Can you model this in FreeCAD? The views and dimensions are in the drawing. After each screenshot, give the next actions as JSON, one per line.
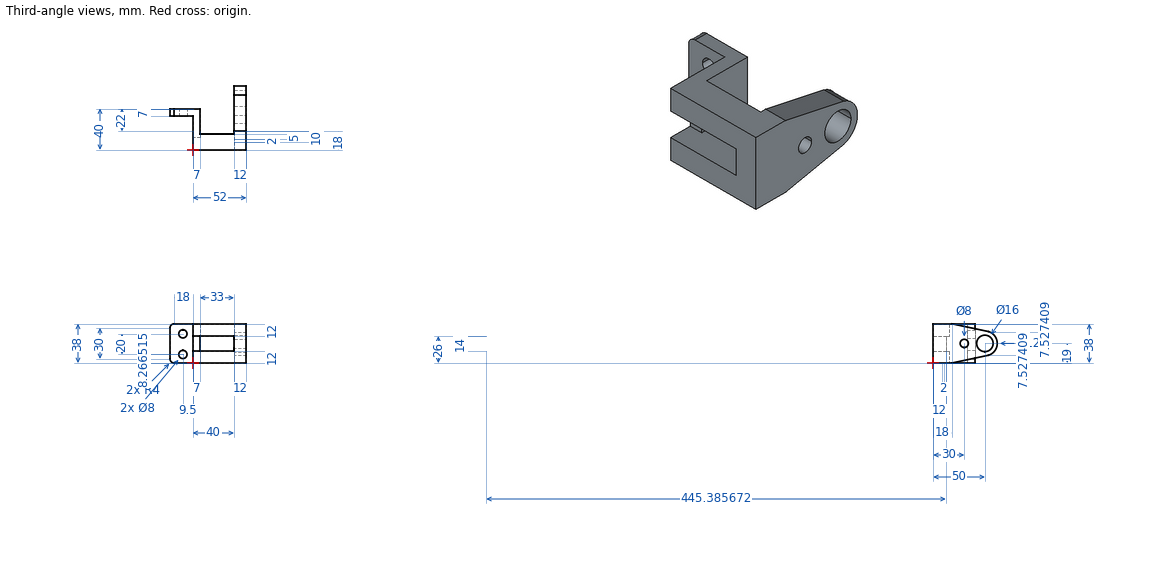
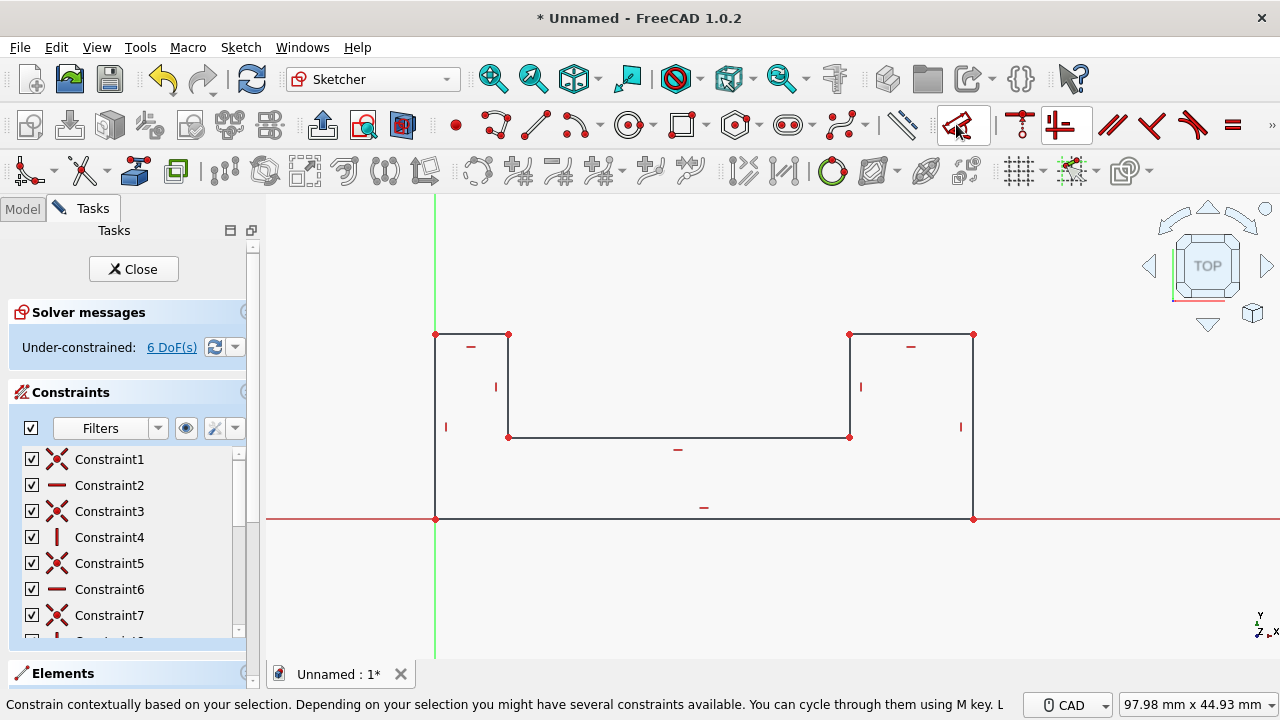
{"action": "left_click", "coordinate": [486, 334]}
{"action": "left_click", "coordinate": [472, 300]}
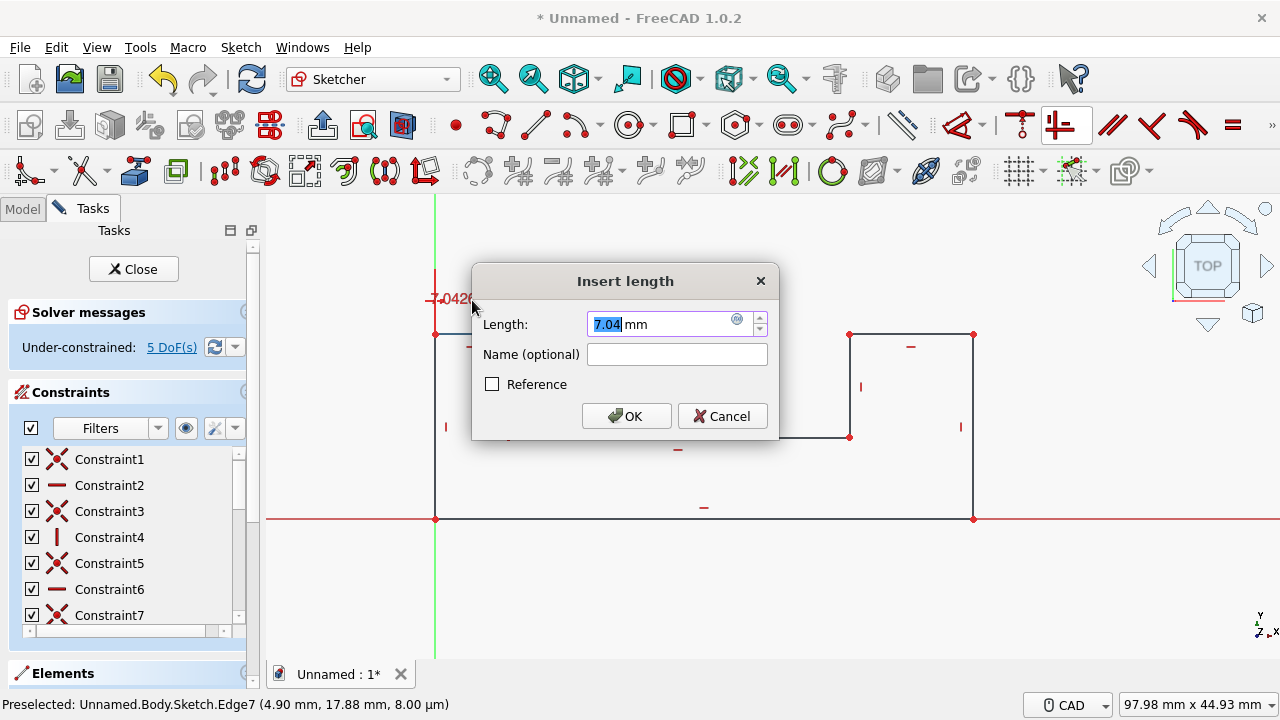
{"action": "type", "text": "7"}
{"action": "key", "text": "Return"}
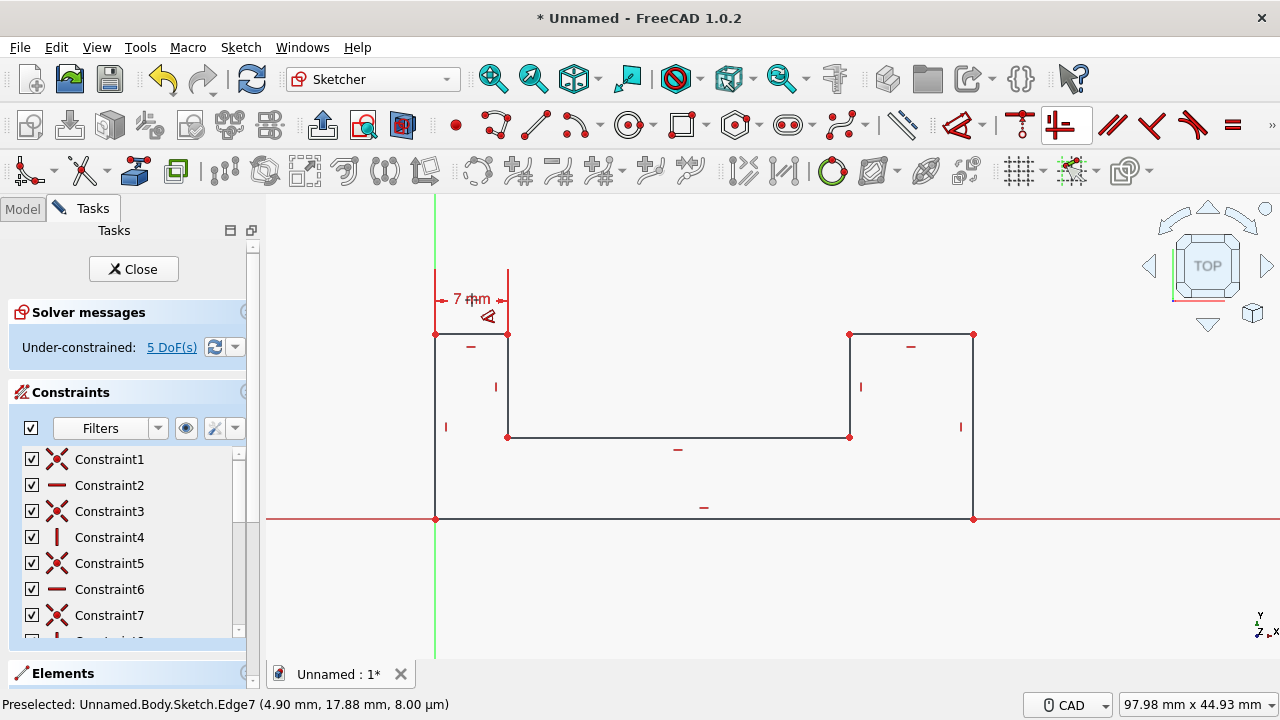
{"action": "left_click", "coordinate": [597, 519]}
{"action": "left_click", "coordinate": [704, 553]}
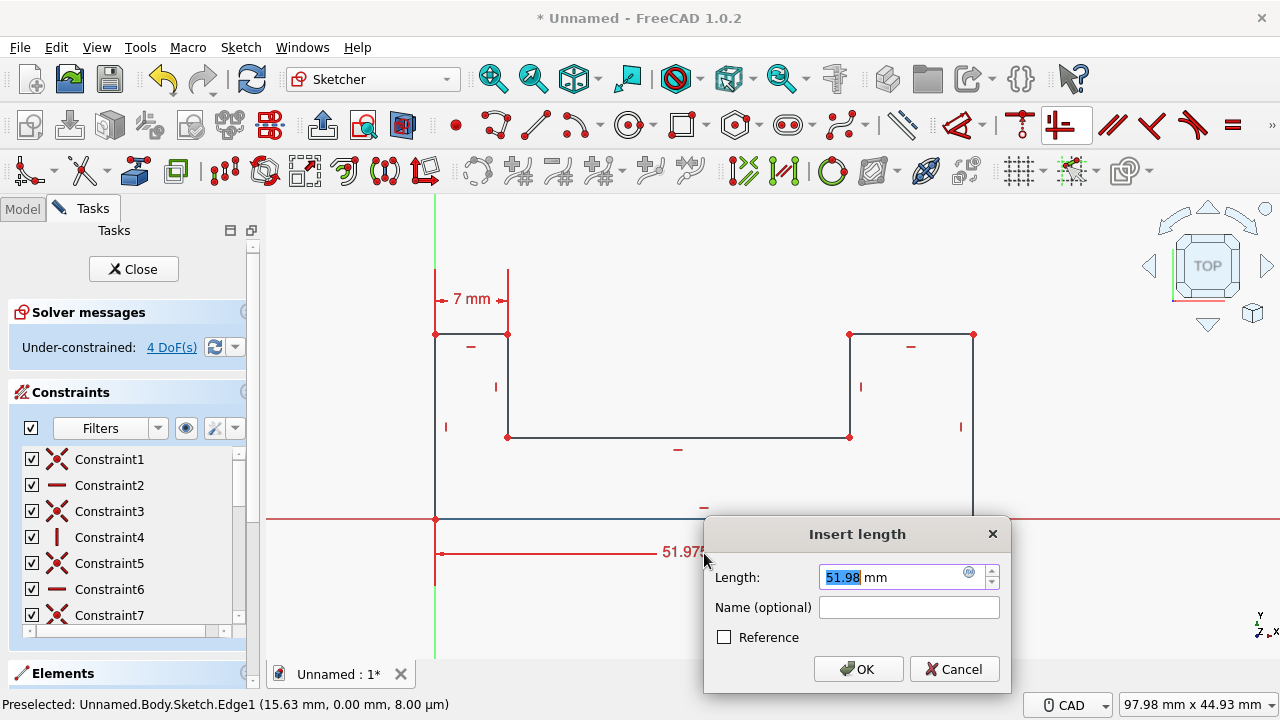
{"action": "type", "text": "52"}
{"action": "key", "text": "Return"}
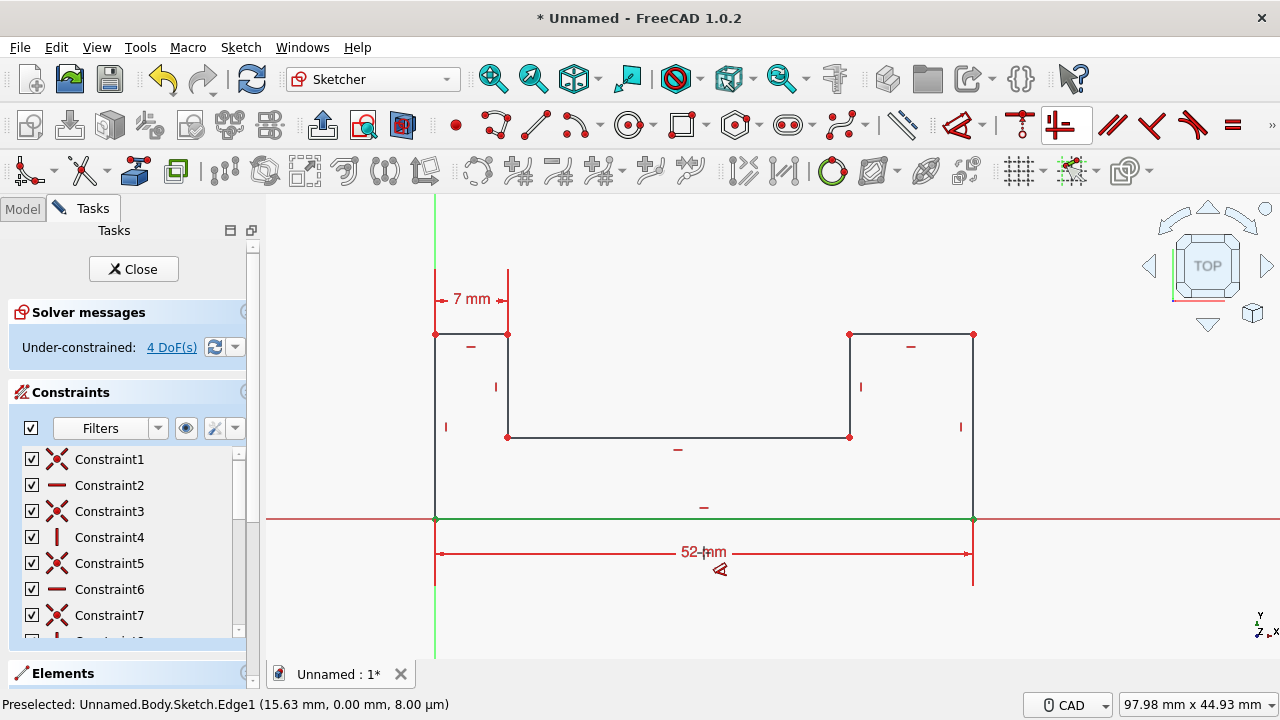
{"action": "left_click", "coordinate": [973, 464]}
{"action": "left_click", "coordinate": [1007, 427]}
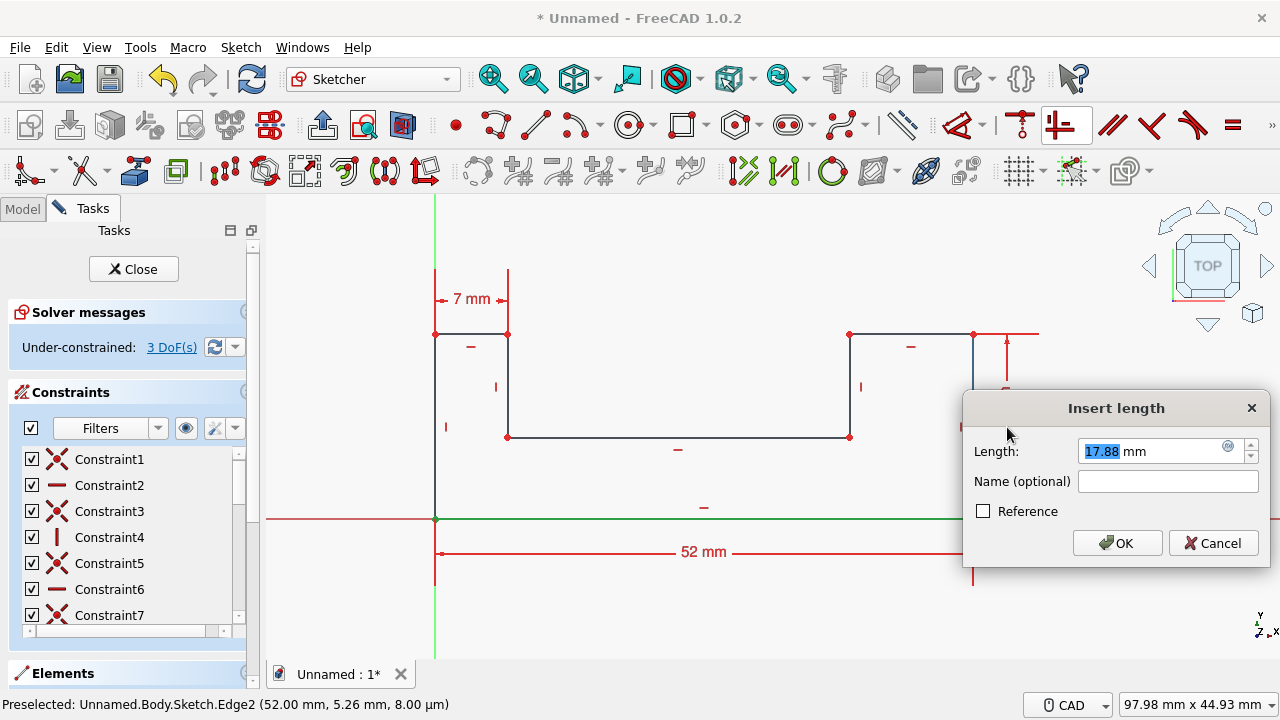
{"action": "type", "text": "18"}
{"action": "key", "text": "Return"}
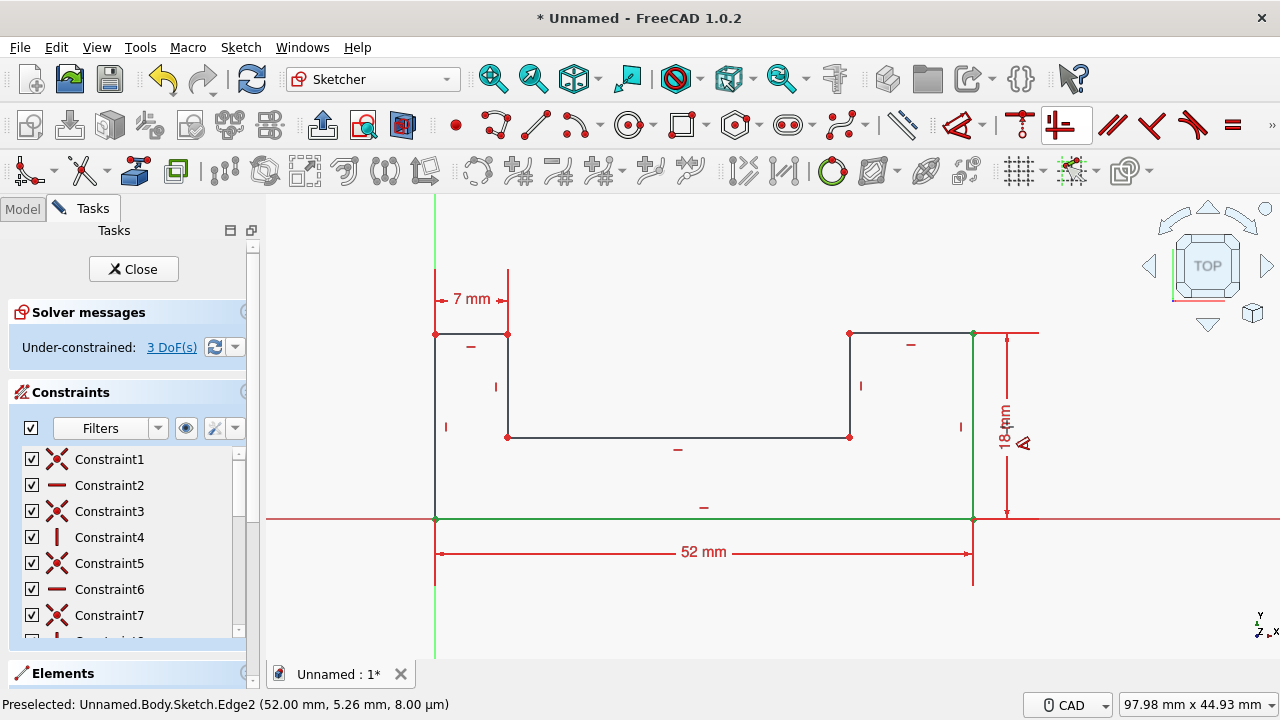
{"action": "left_click", "coordinate": [936, 333]}
{"action": "left_click", "coordinate": [912, 299]}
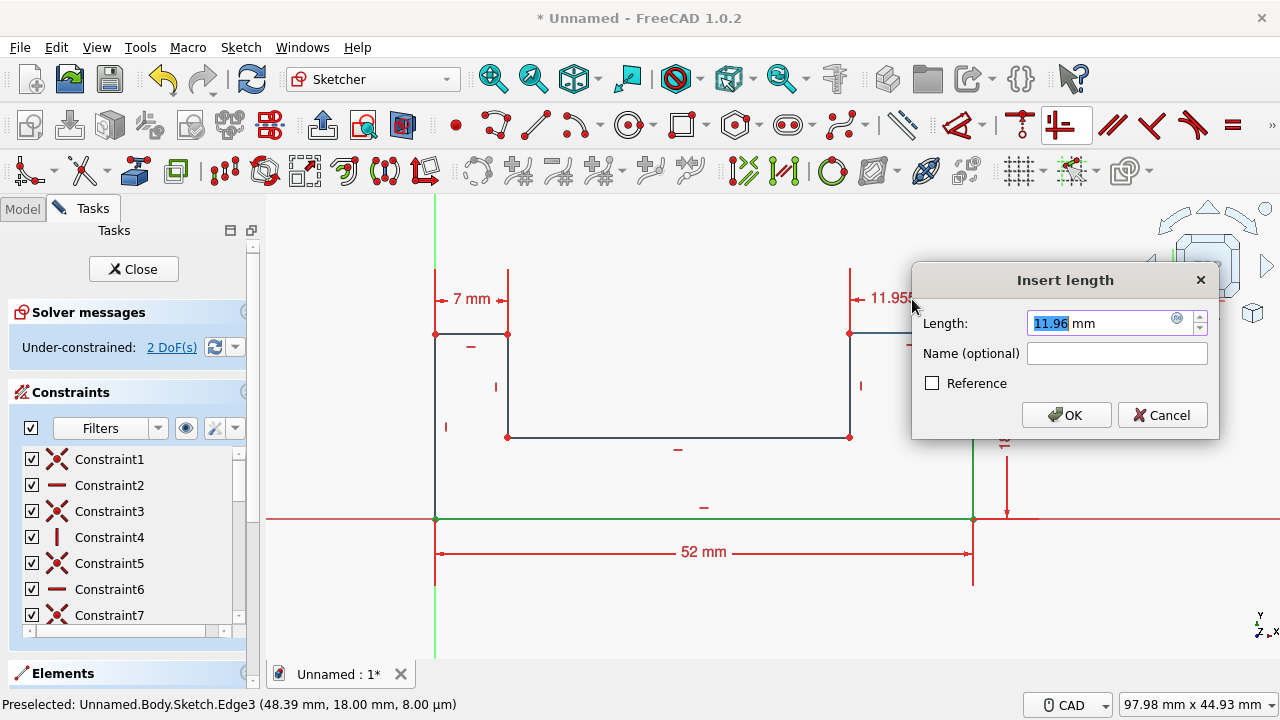
{"action": "type", "text": "12"}
{"action": "key", "text": "Return"}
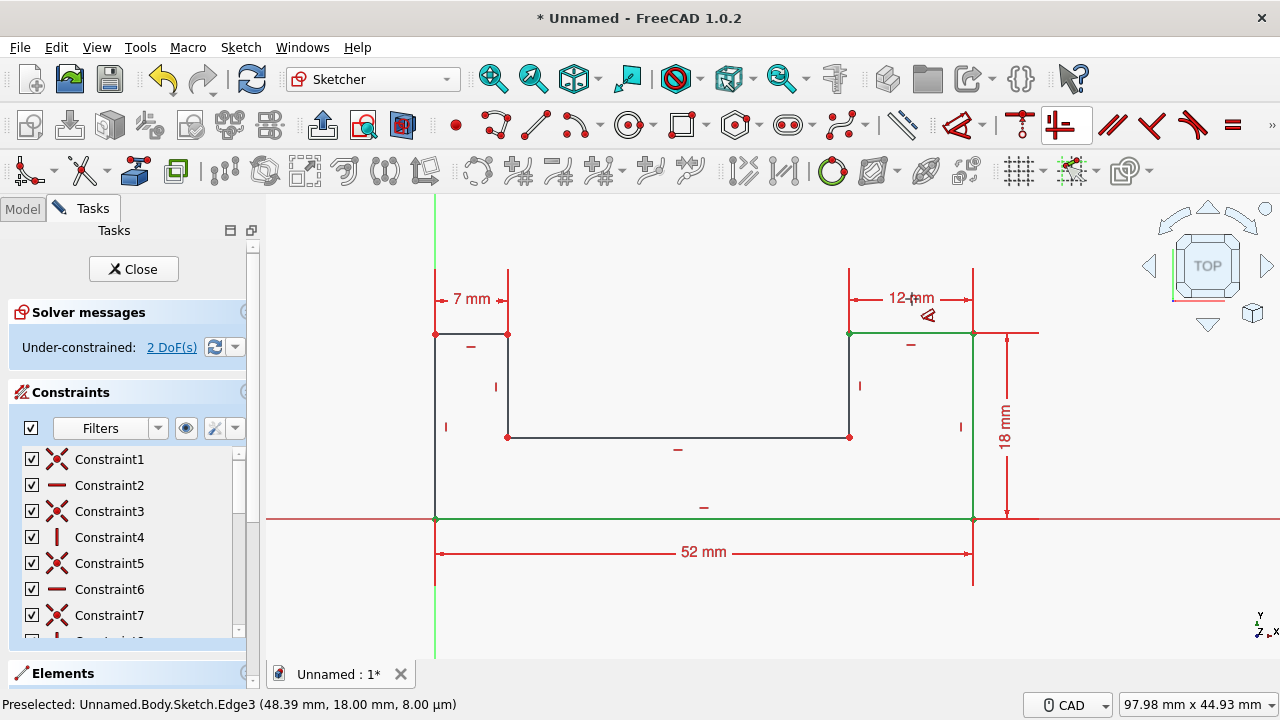
{"action": "left_click", "coordinate": [849, 365]}
{"action": "left_click", "coordinate": [883, 386]}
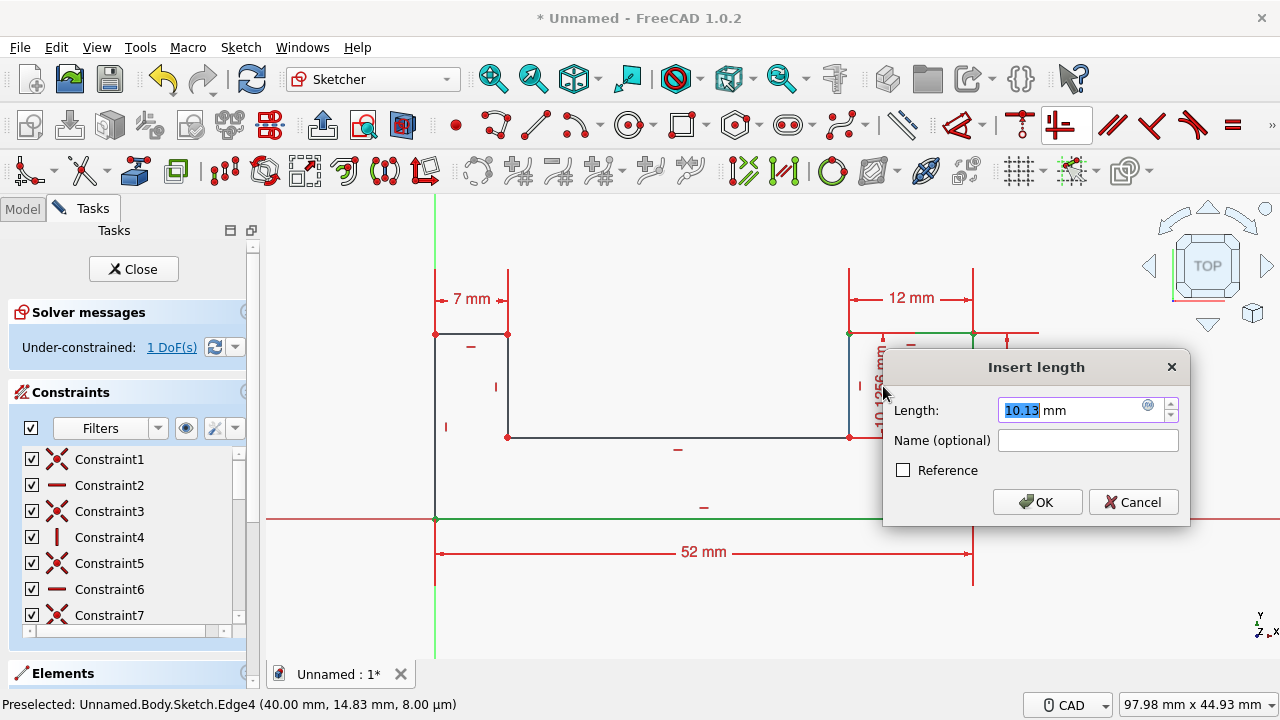
{"action": "type", "text": "10"}
{"action": "key", "text": "Return"}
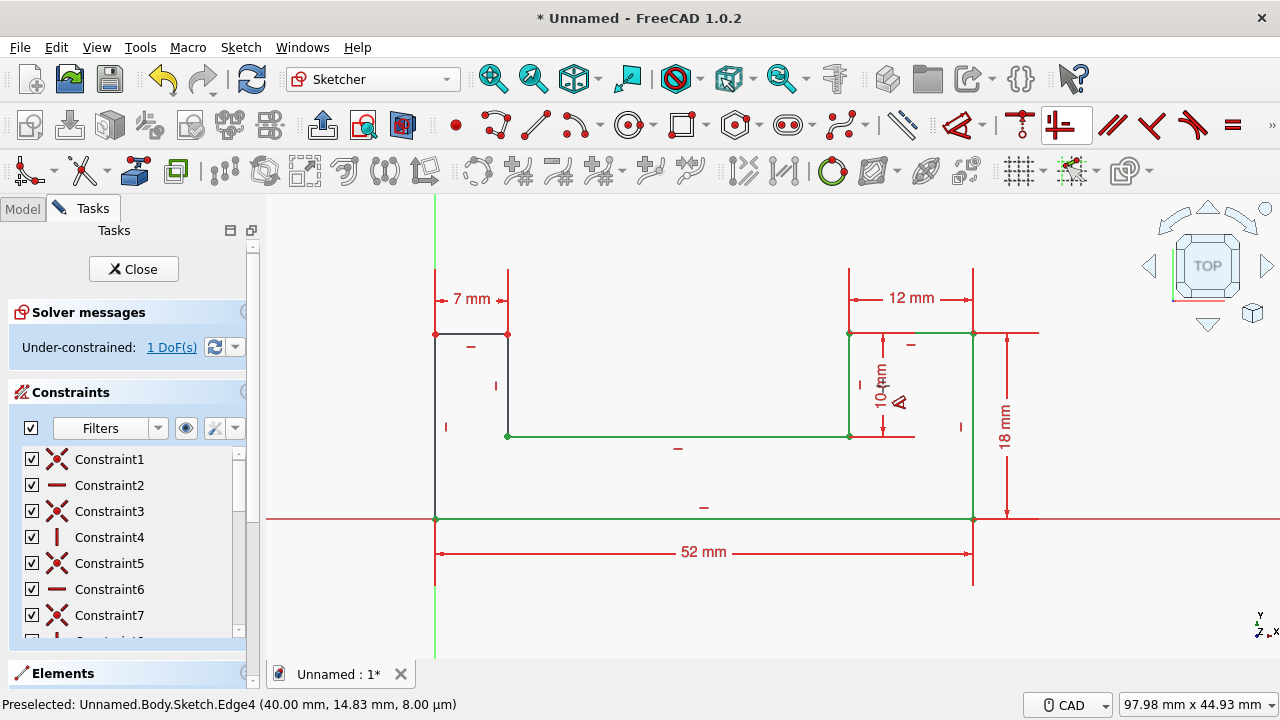
{"action": "left_click", "coordinate": [508, 406]}
{"action": "left_click", "coordinate": [474, 386]}